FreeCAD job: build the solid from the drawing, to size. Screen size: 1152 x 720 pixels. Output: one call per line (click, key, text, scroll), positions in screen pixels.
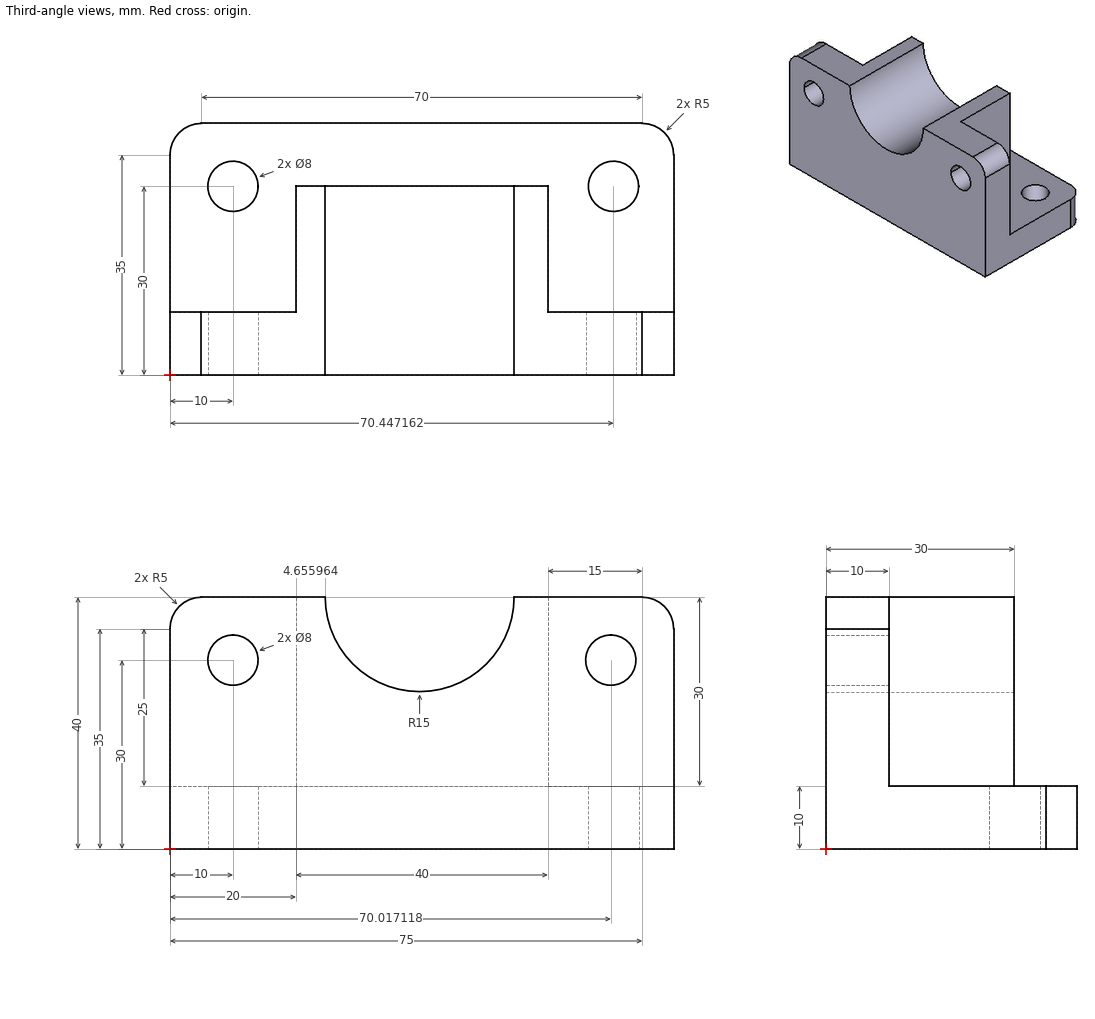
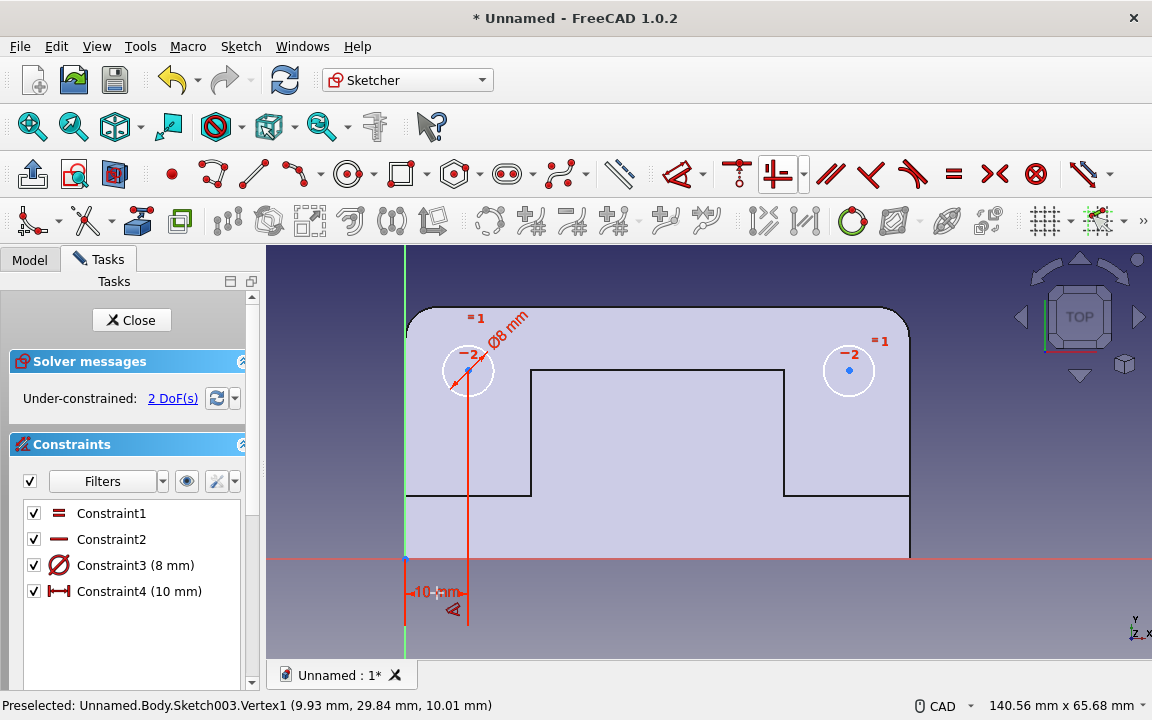
click(468, 371)
click(371, 465)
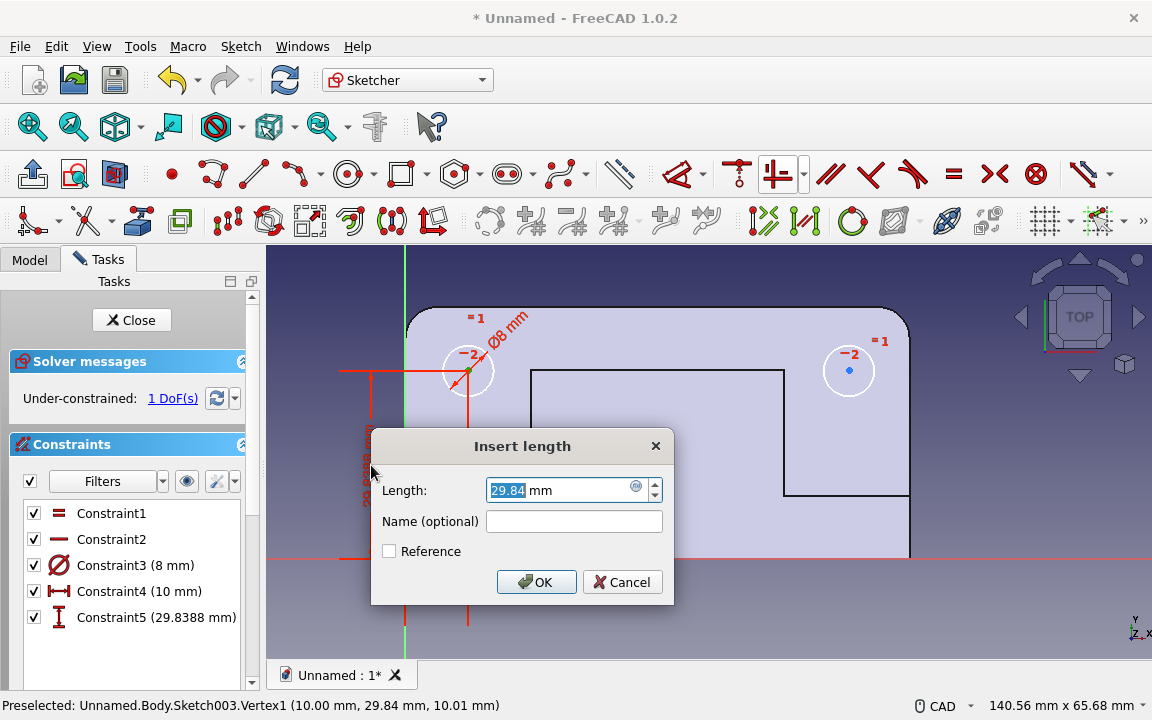
text(30)
key(Return)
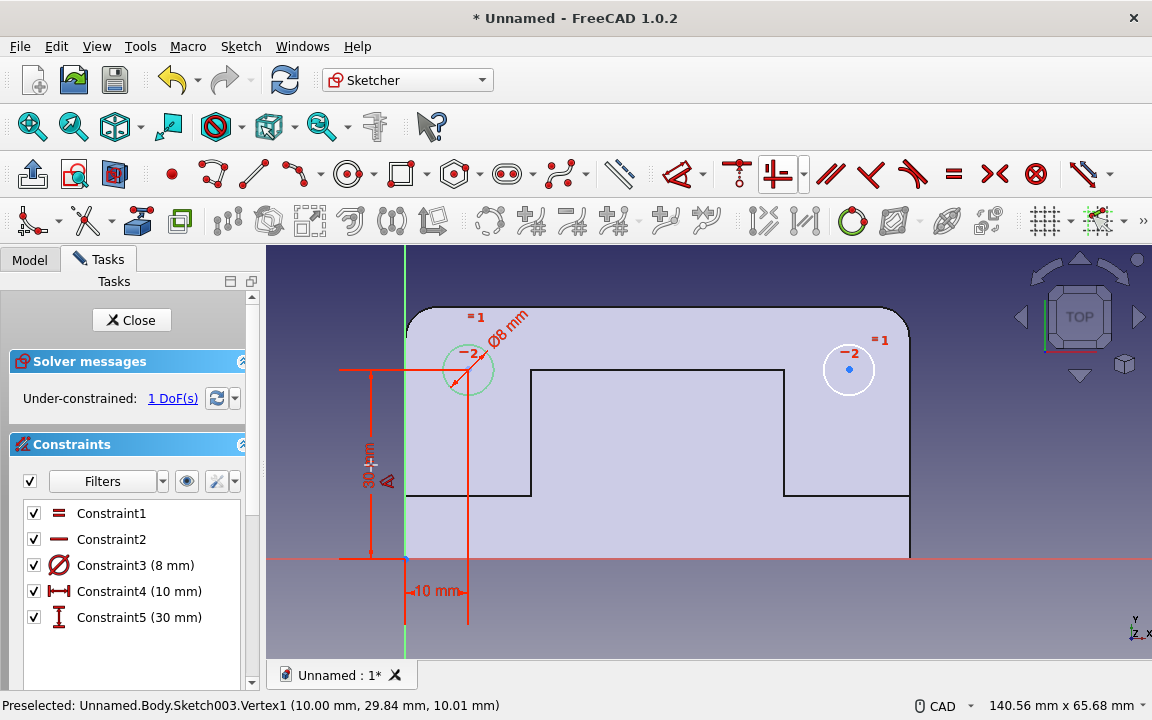
click(849, 370)
click(627, 593)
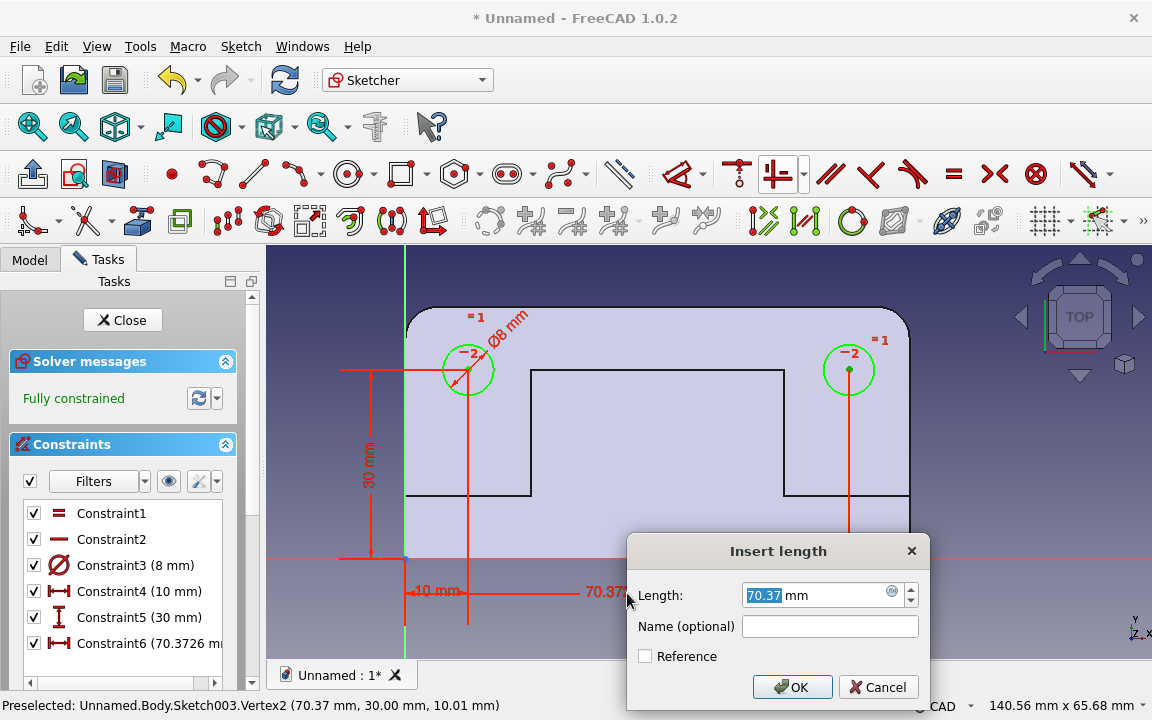
text(70.447162)
key(Return)
key(Escape)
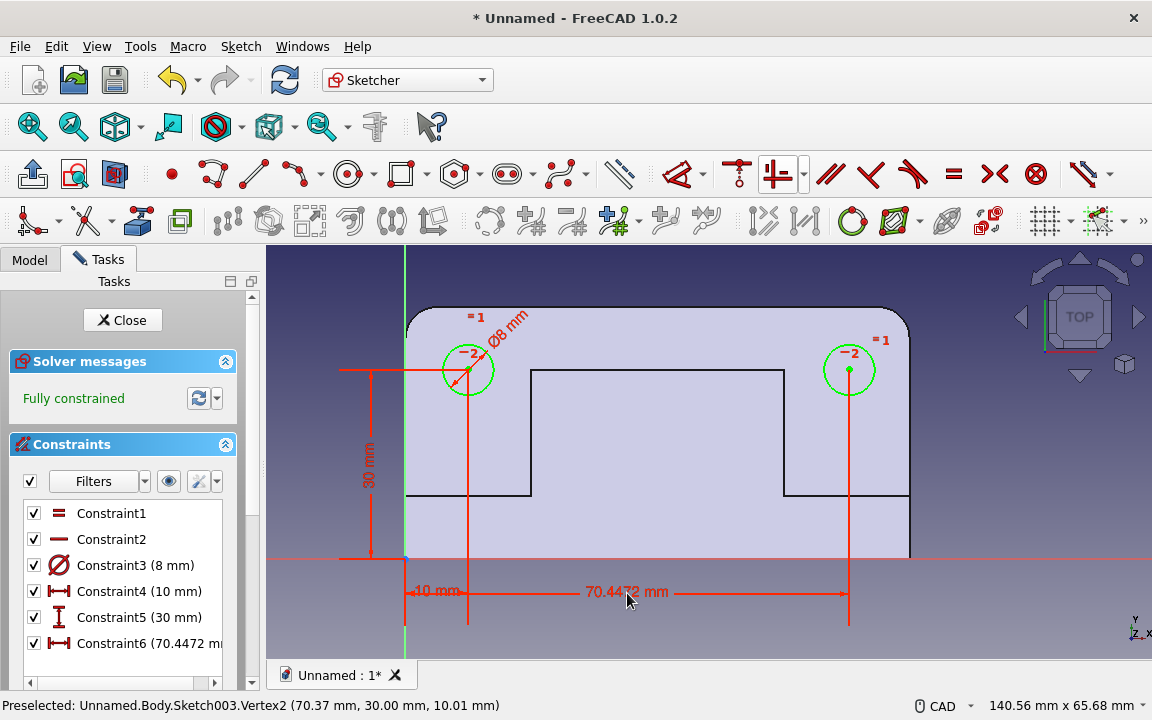
click(123, 320)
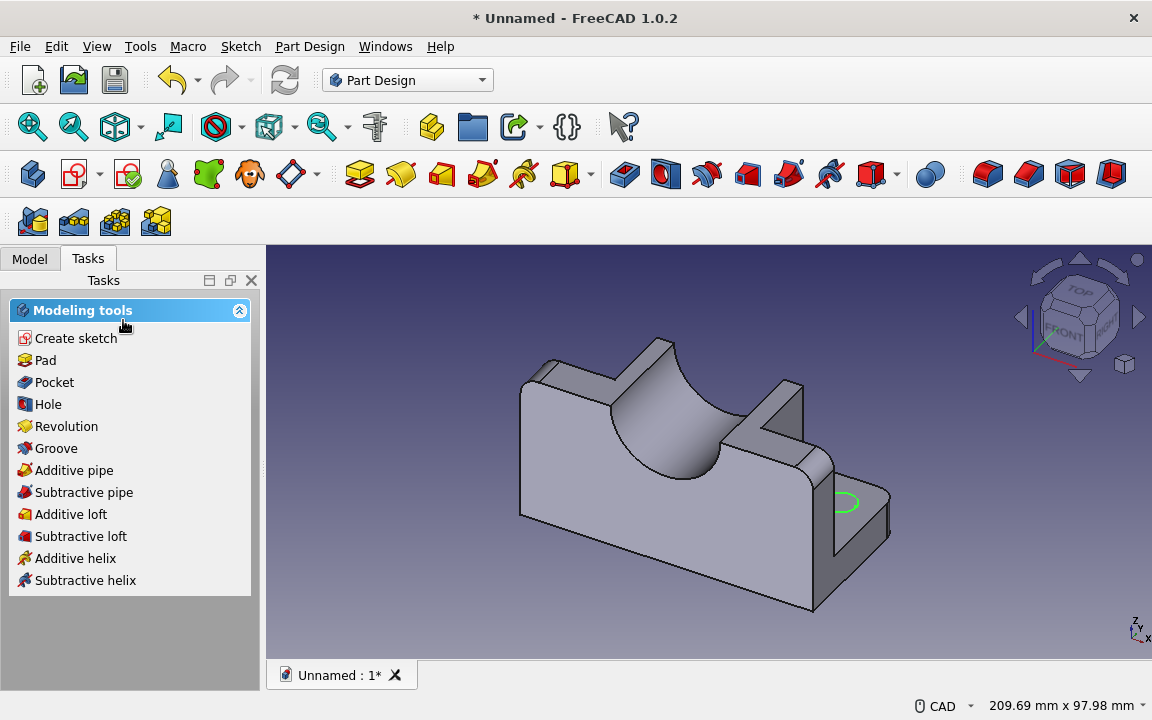
click(625, 174)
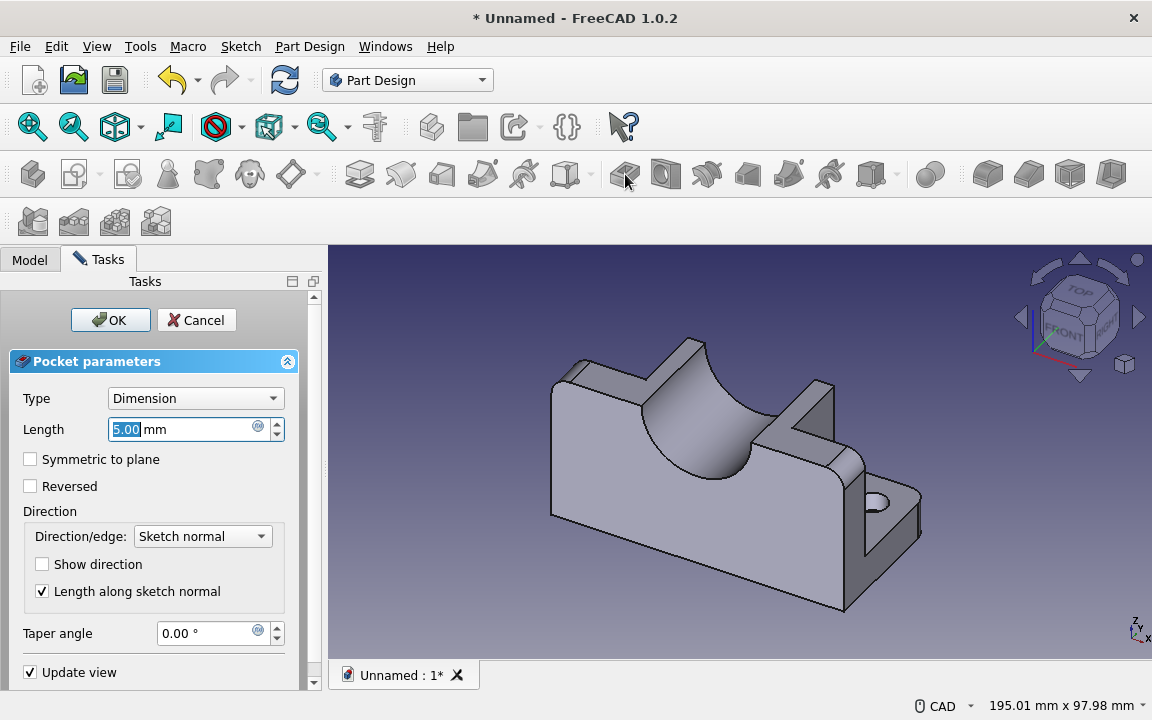
text(10)
key(Tab)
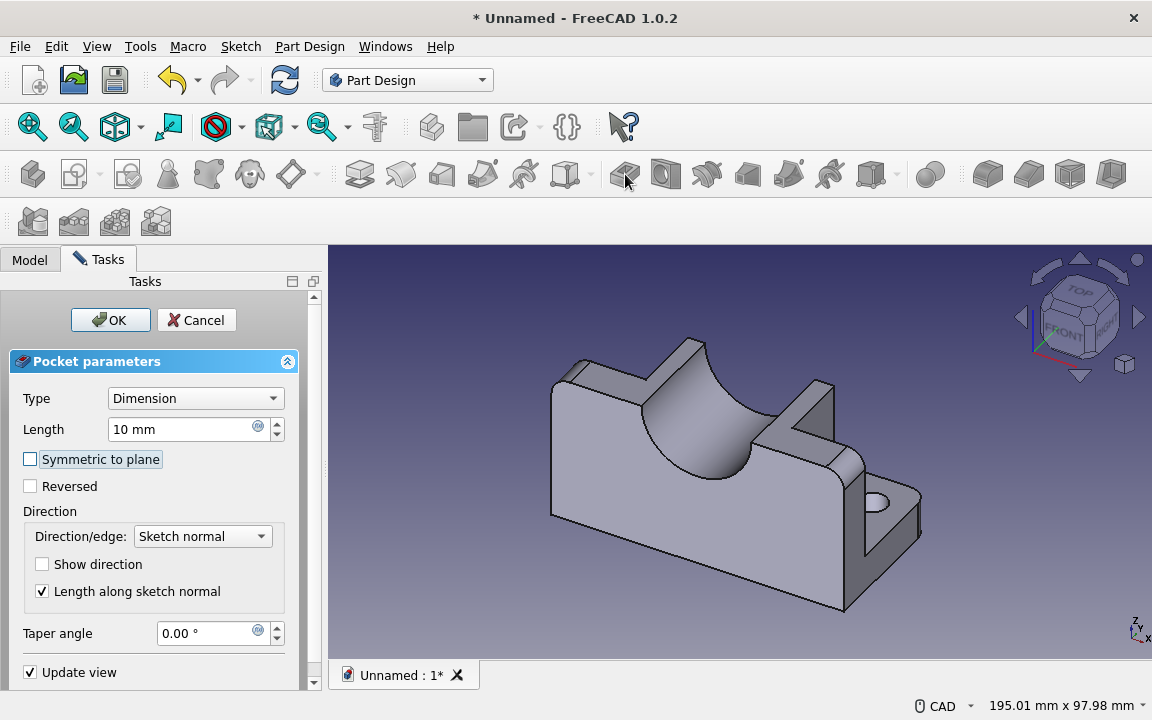
click(111, 320)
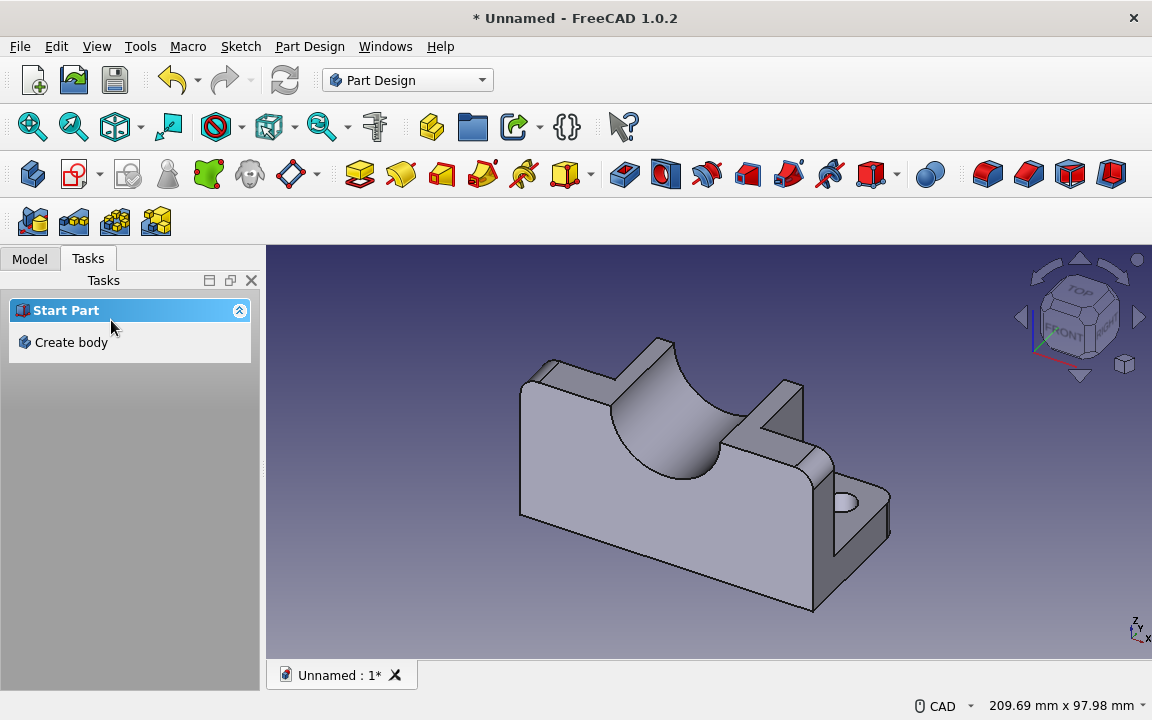
key(4)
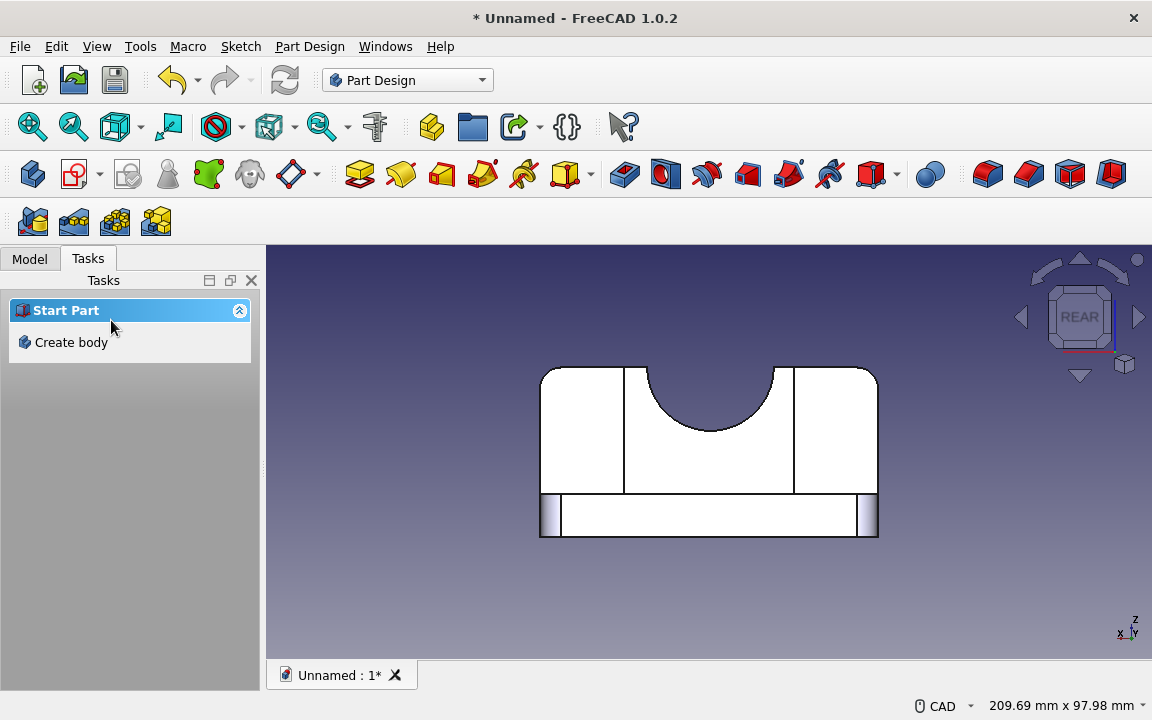
key(v)
key(f)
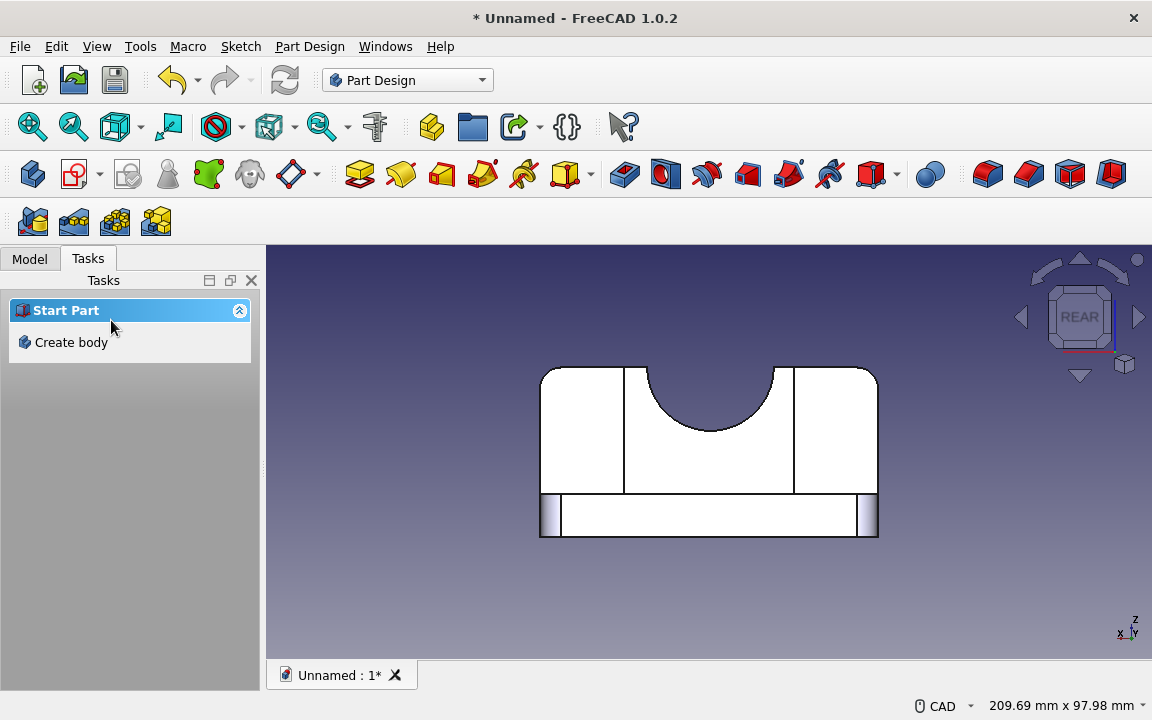
click(836, 412)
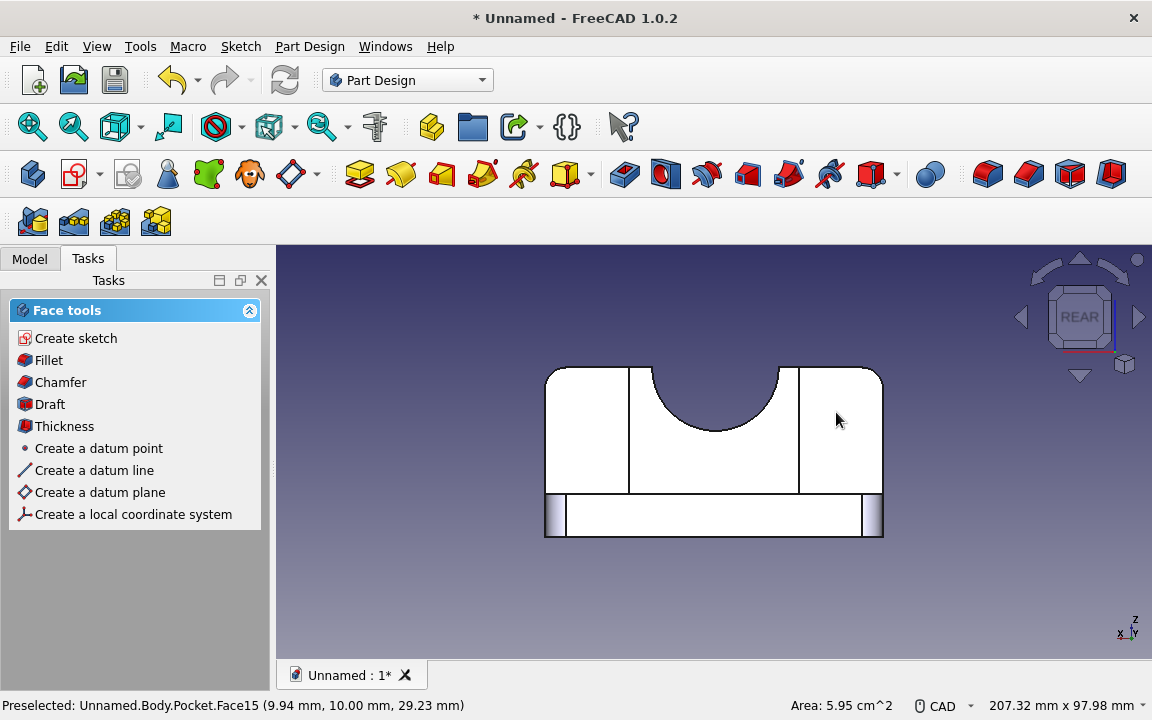
click(74, 174)